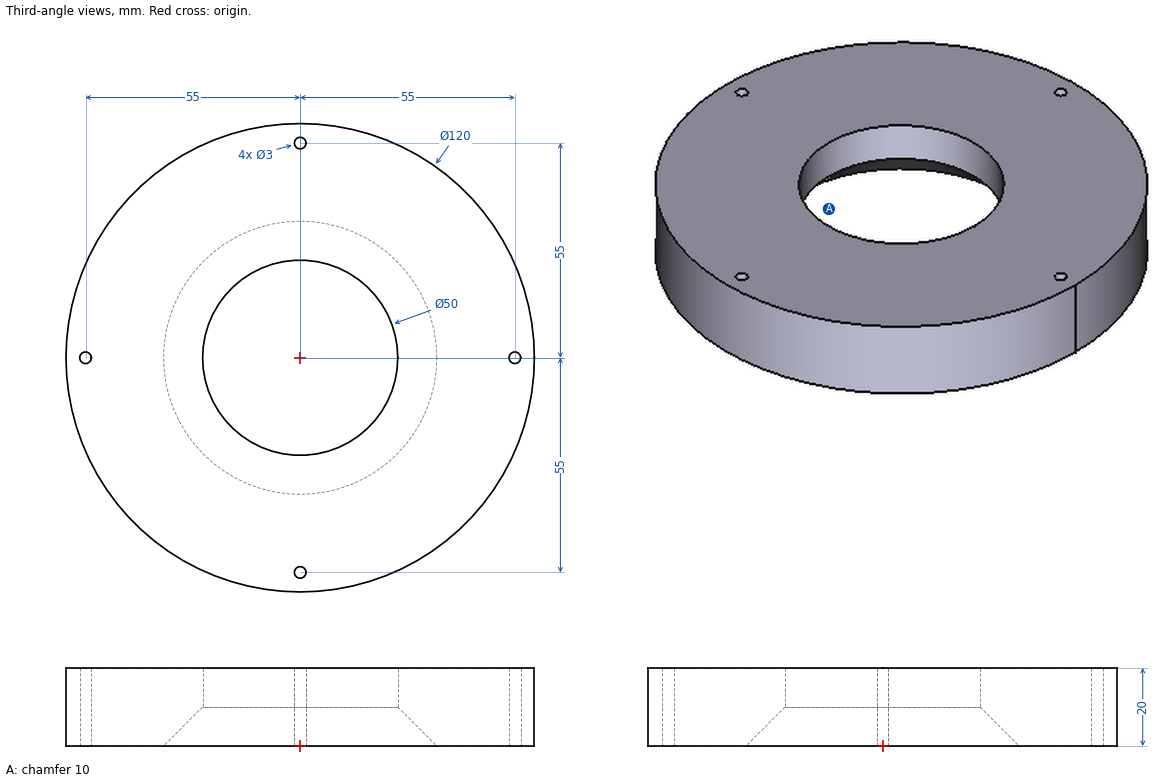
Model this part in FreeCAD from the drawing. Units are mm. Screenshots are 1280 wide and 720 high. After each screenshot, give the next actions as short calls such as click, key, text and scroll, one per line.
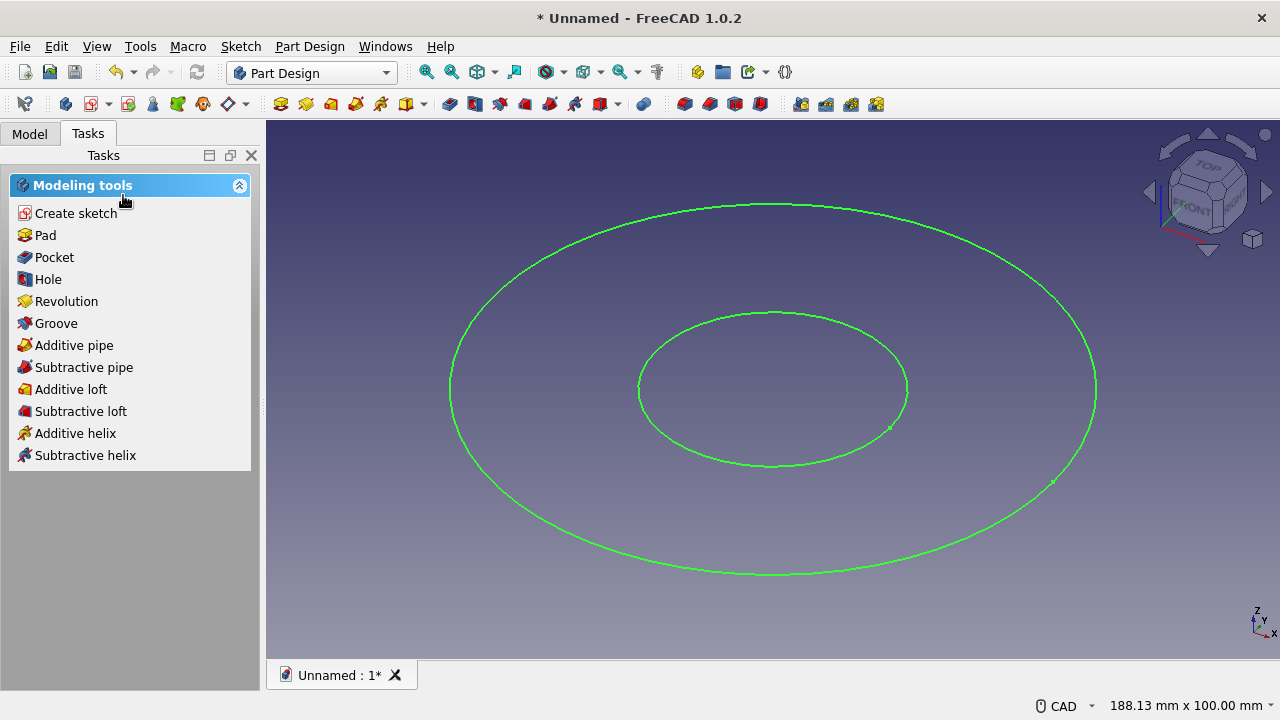
click(281, 104)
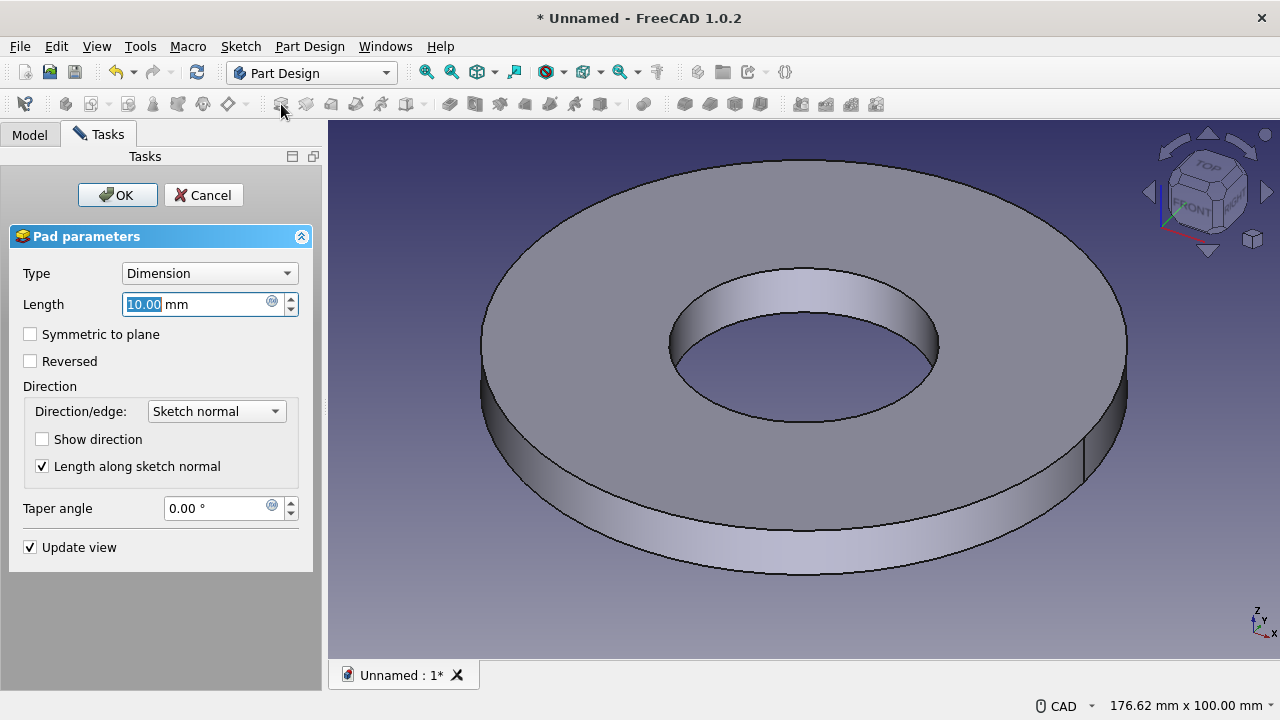
text(20)
key(Tab)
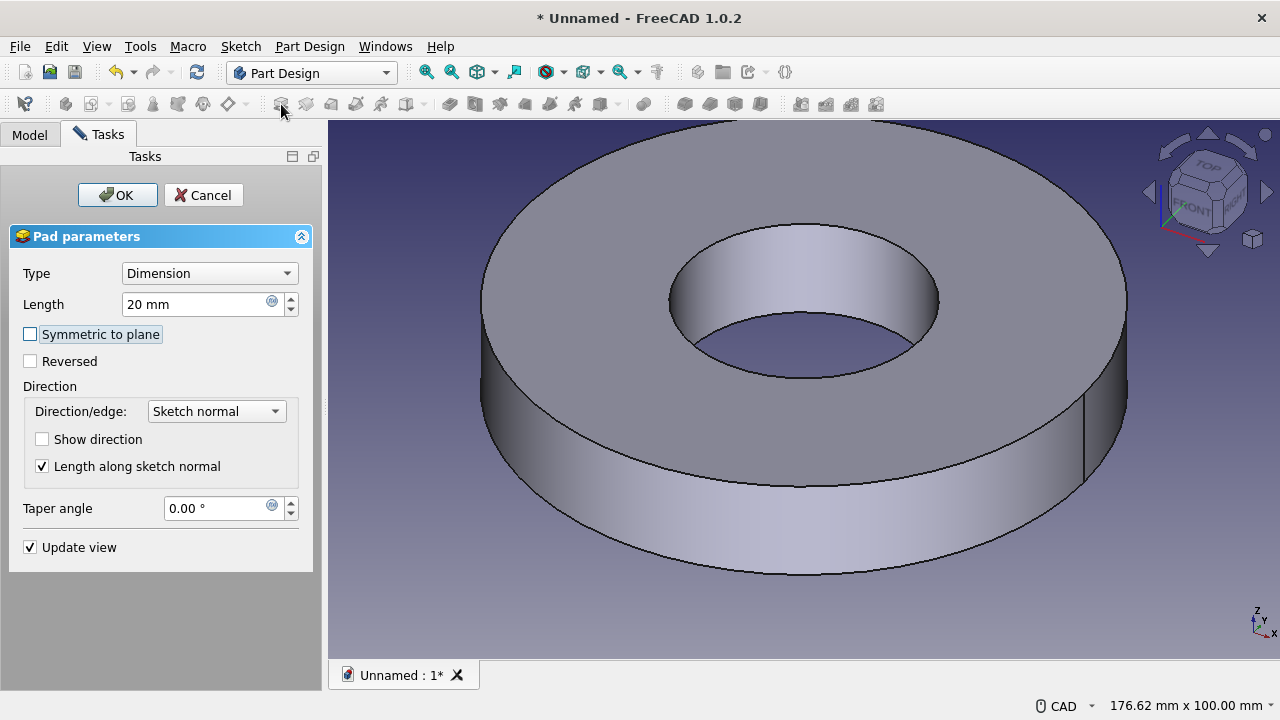
click(118, 195)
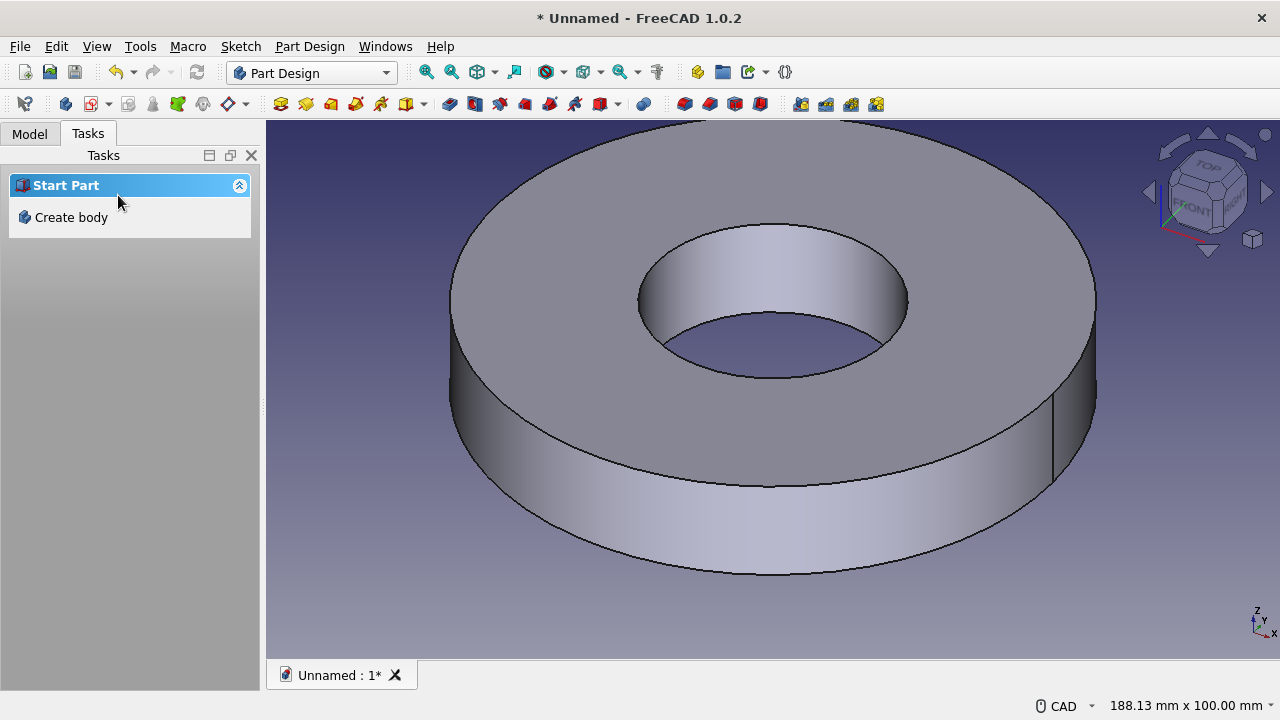
click(427, 72)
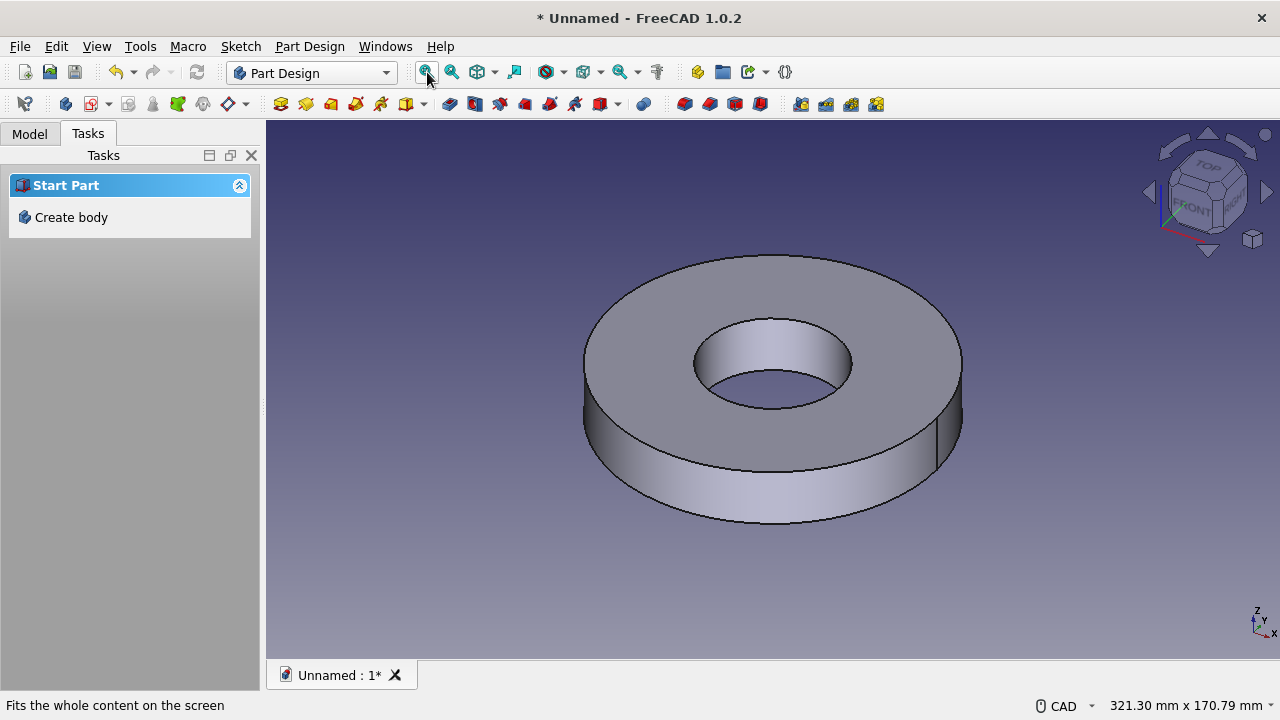
key(0)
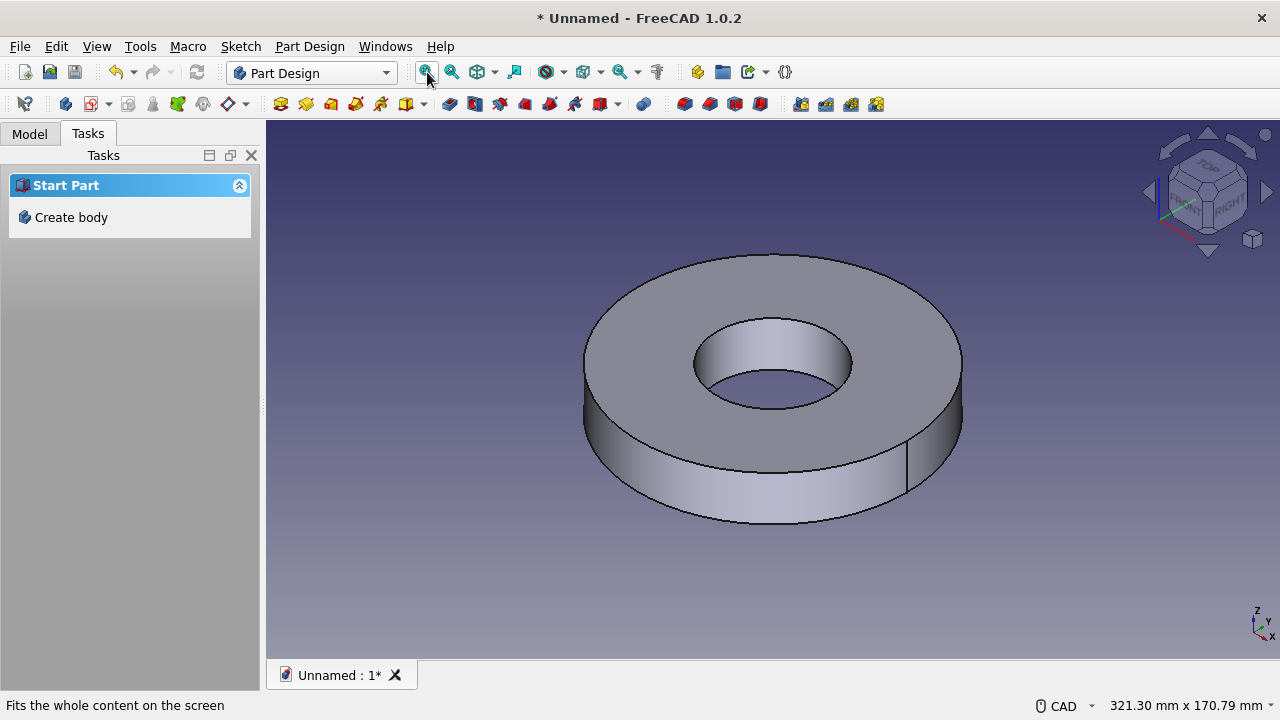
key(2)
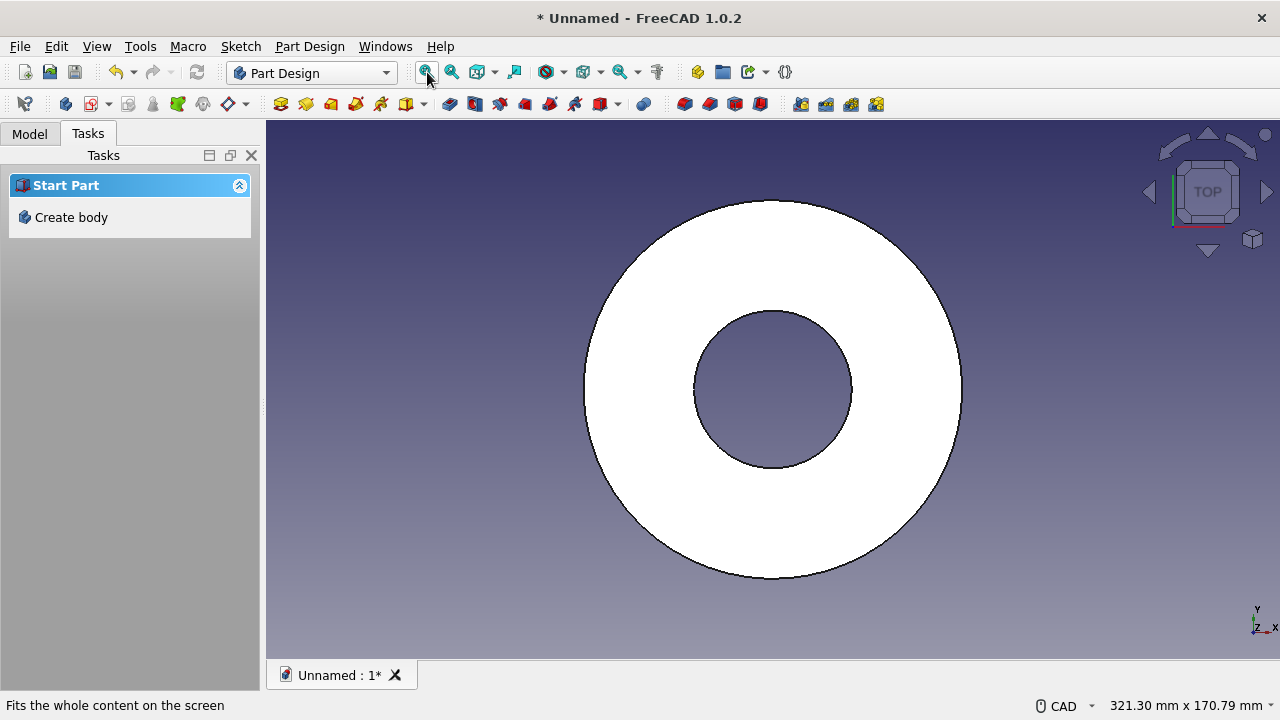
key(1)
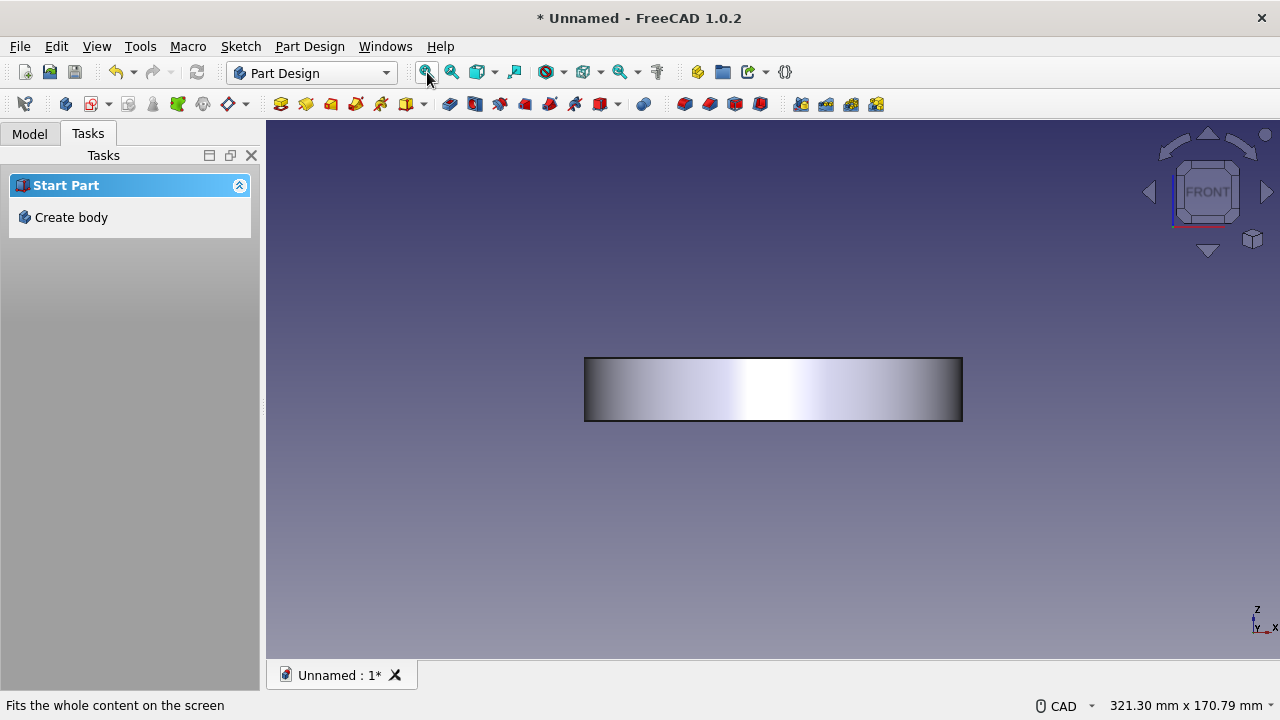
key(v)
key(f)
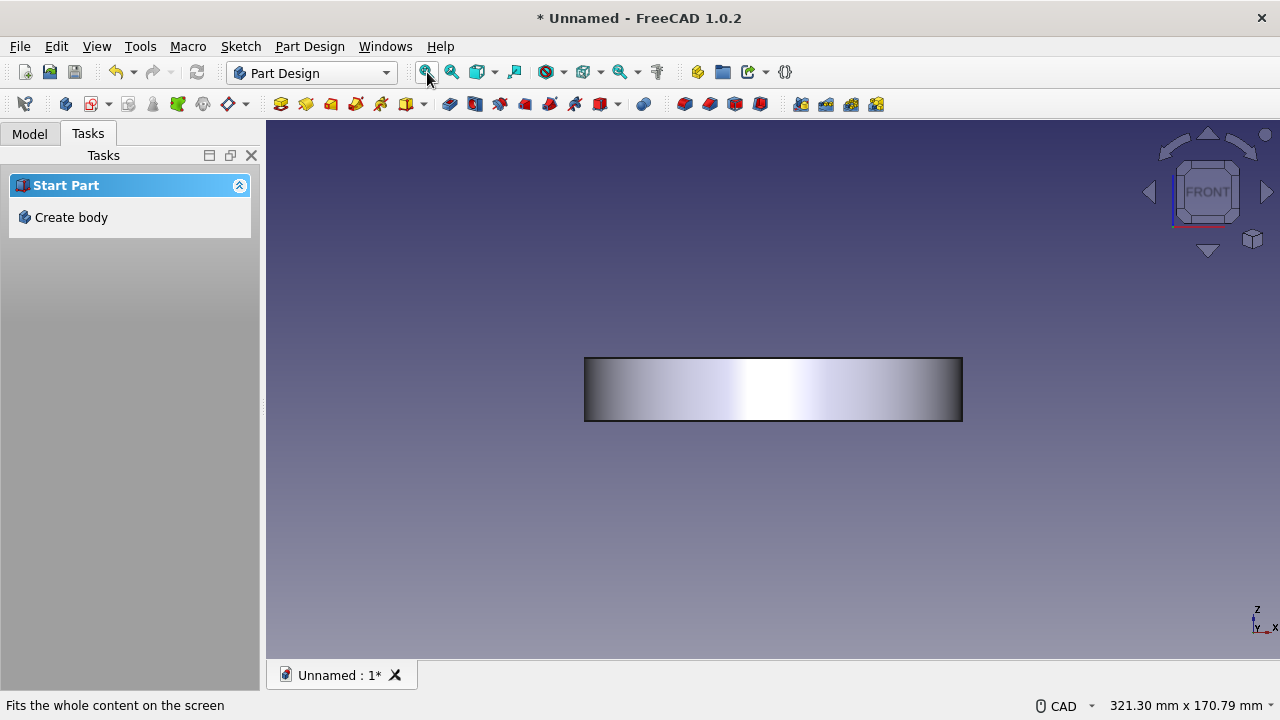
key(3)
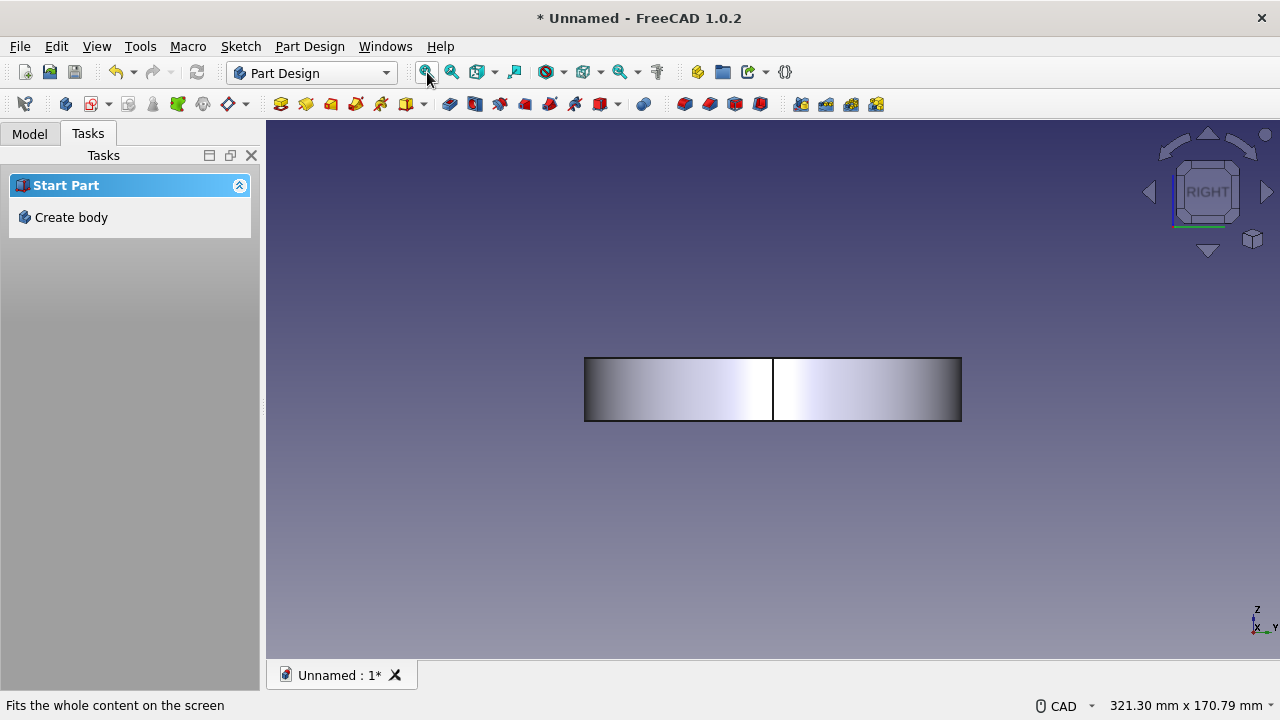
key(v)
key(f)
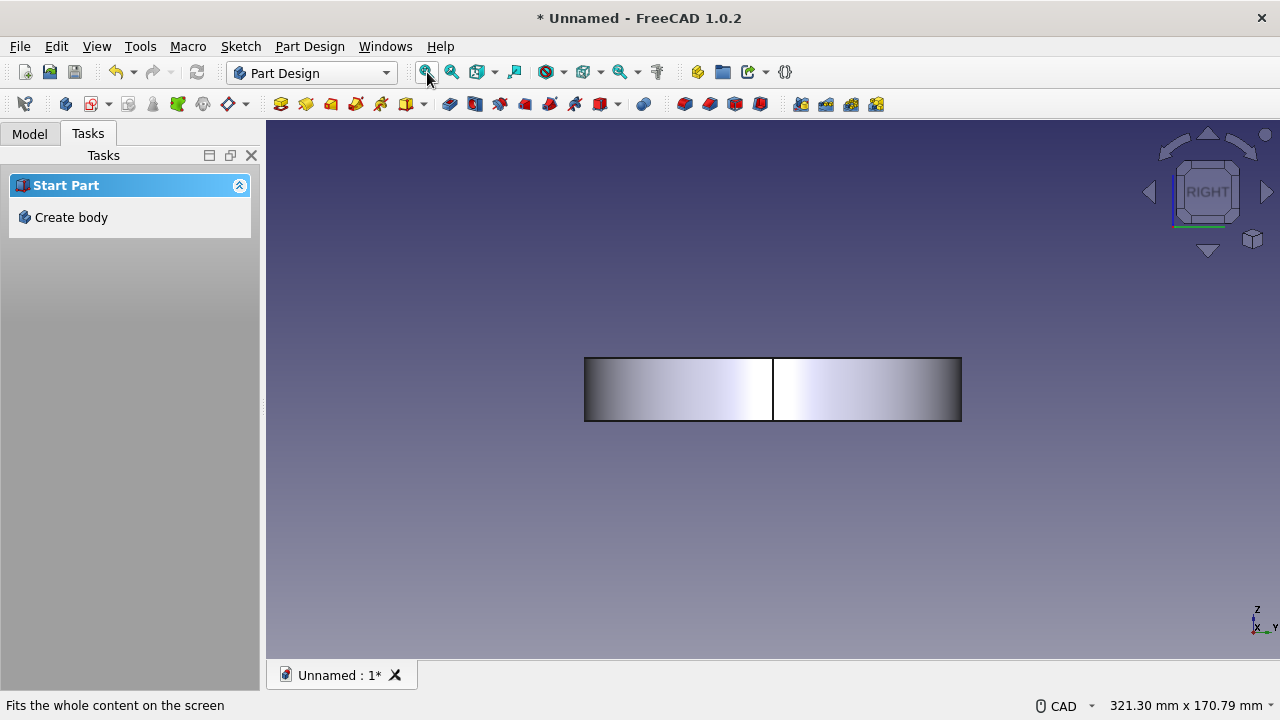
key(5)